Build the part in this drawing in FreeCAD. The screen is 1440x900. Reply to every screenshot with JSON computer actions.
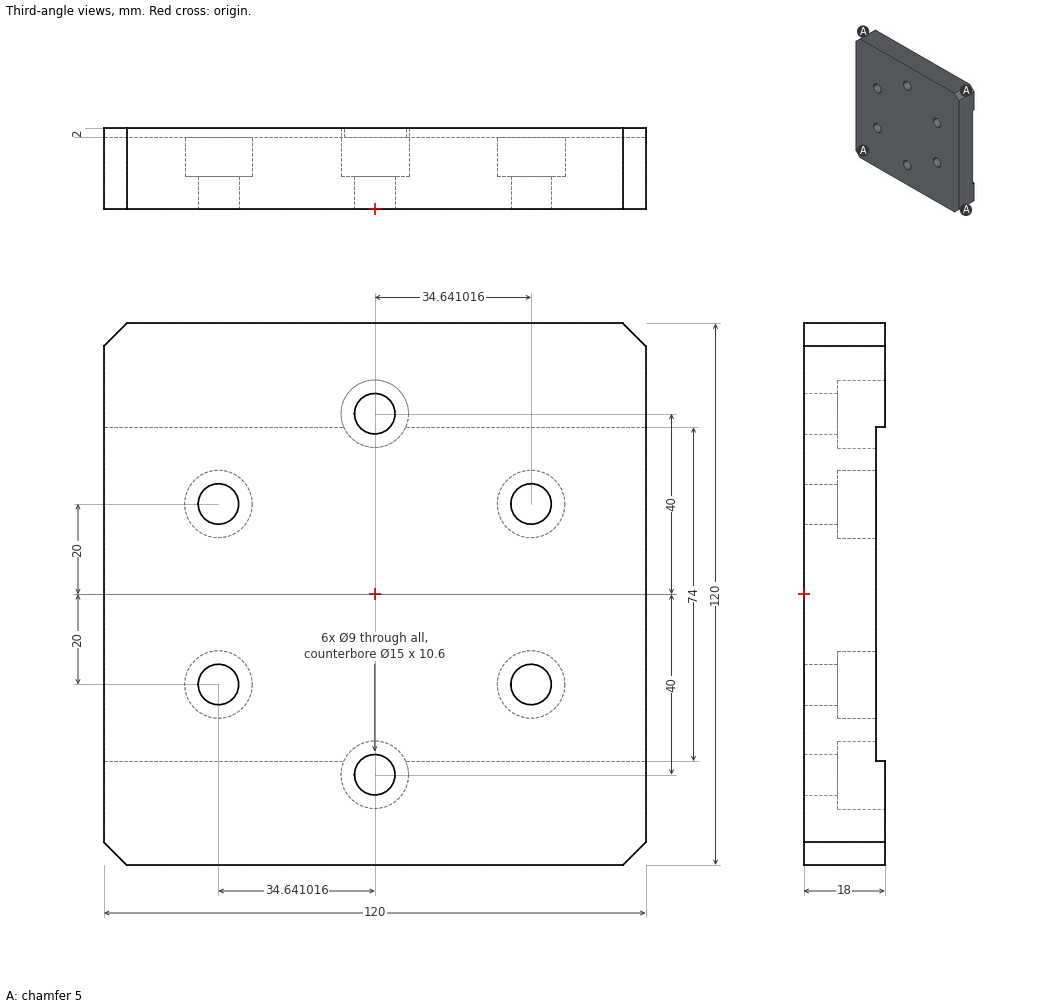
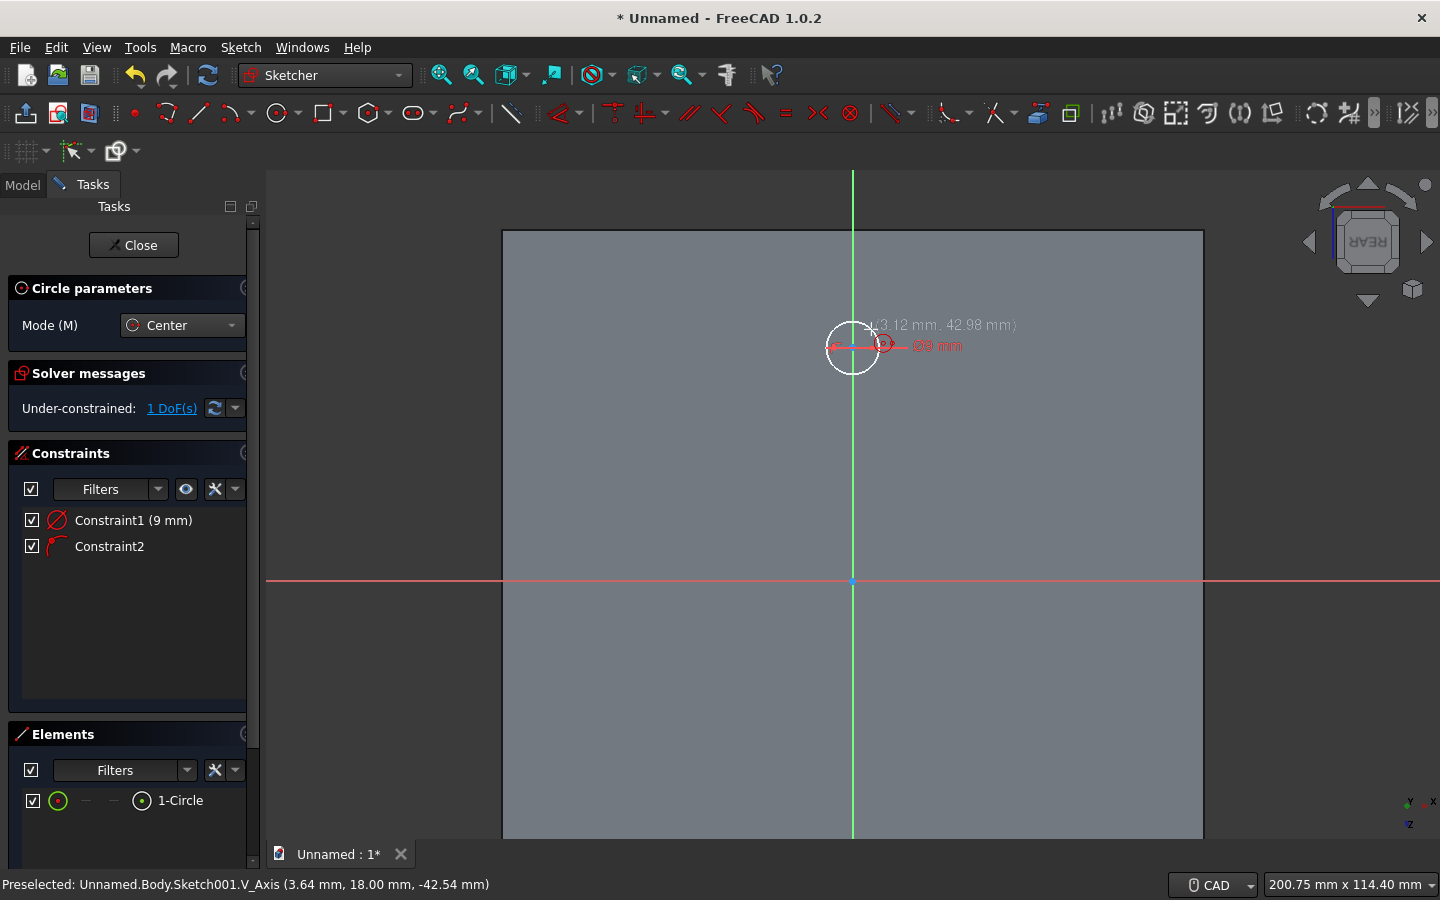
{"action": "left_click", "coordinate": [650, 464]}
{"action": "mouse_move", "coordinate": [669, 446]}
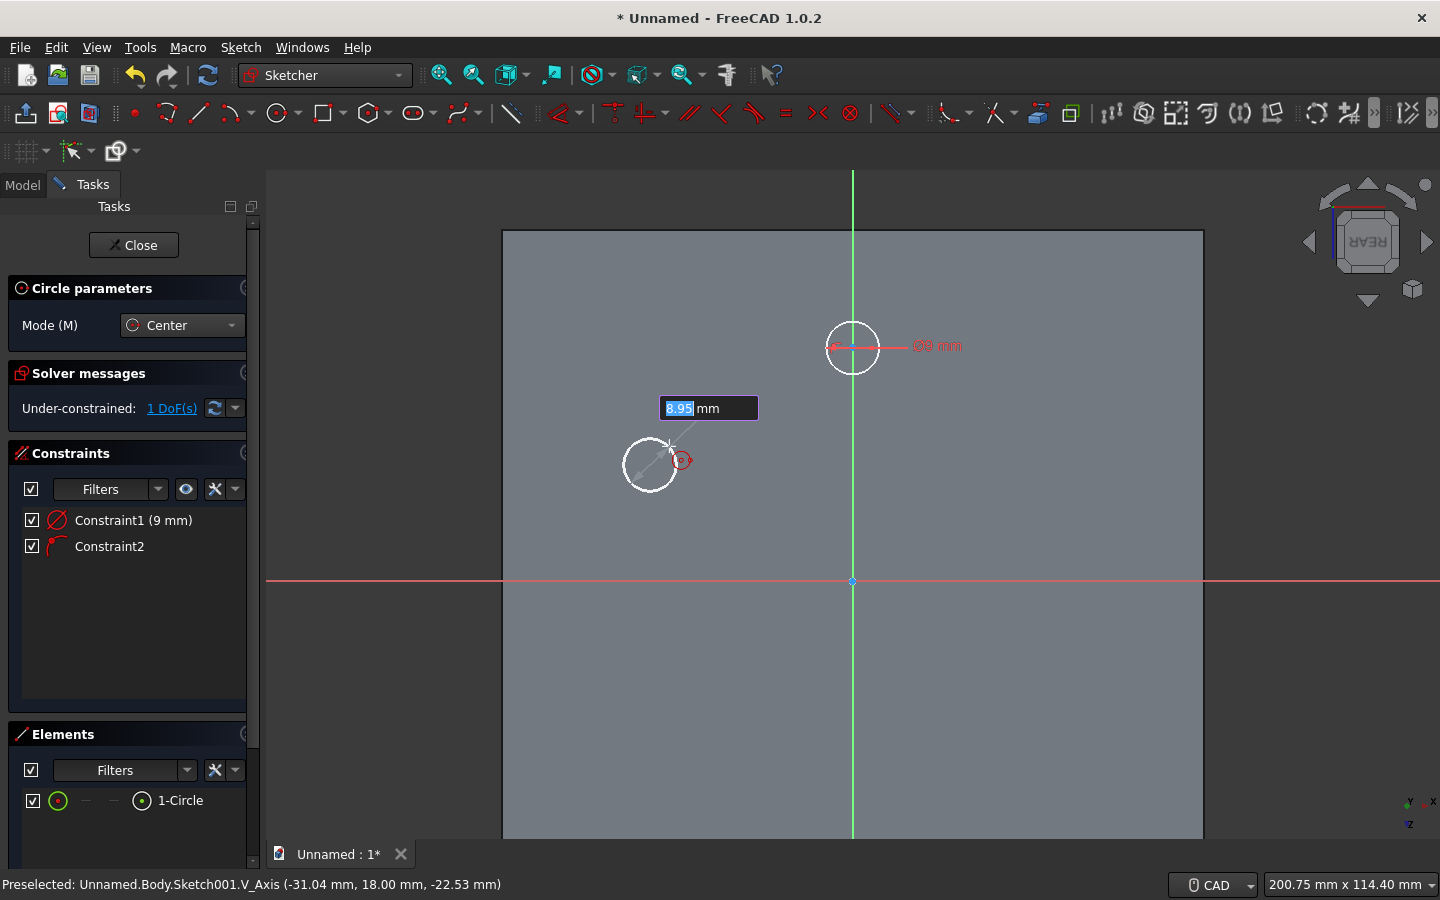
{"action": "type", "text": "9"}
{"action": "key", "text": "Return"}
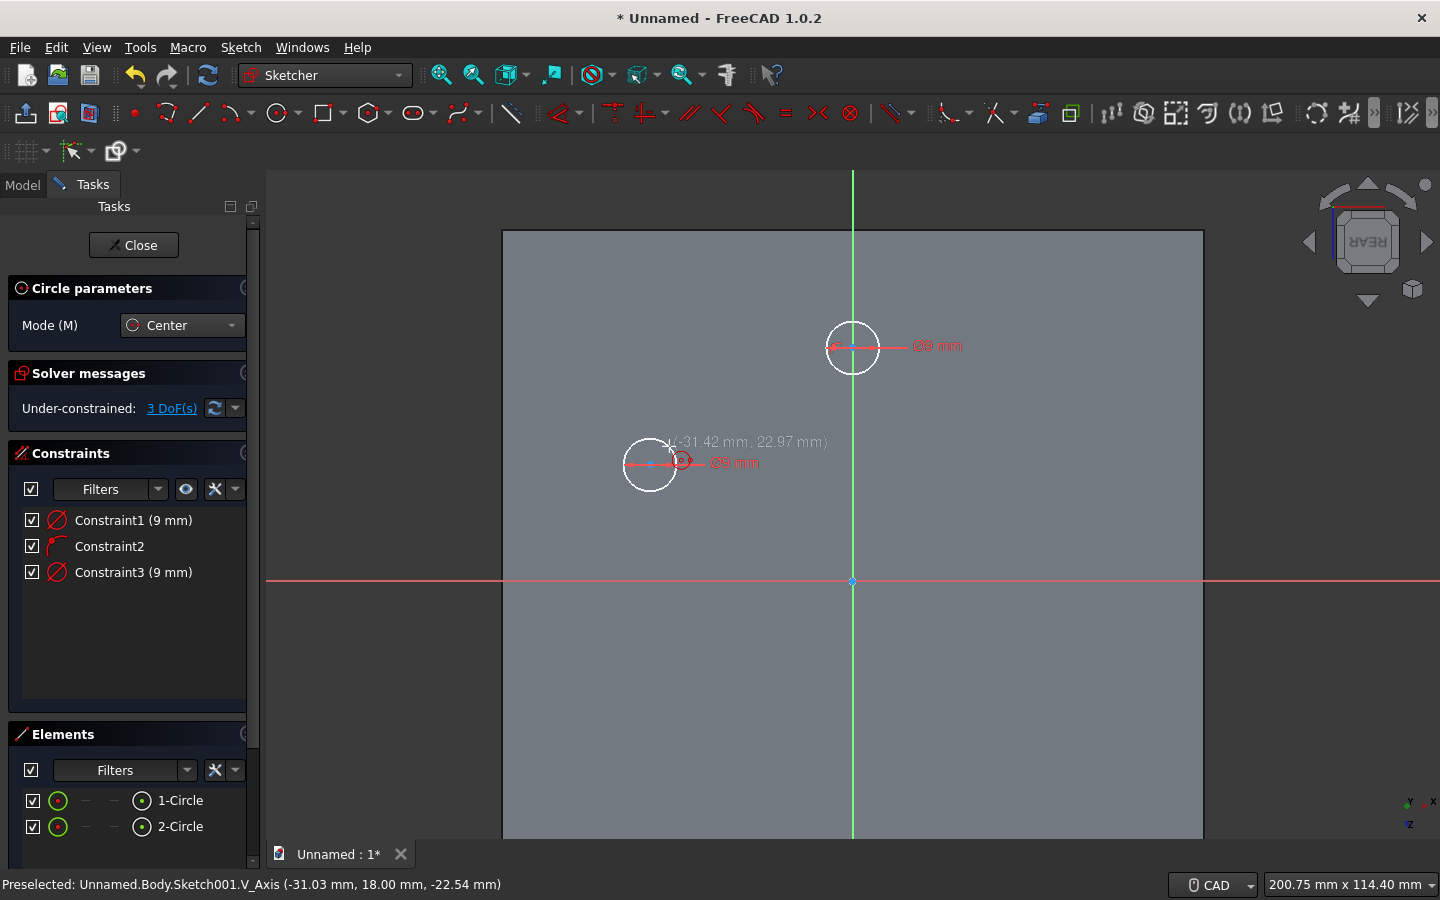
{"action": "left_click", "coordinate": [650, 698]}
{"action": "mouse_move", "coordinate": [669, 680]}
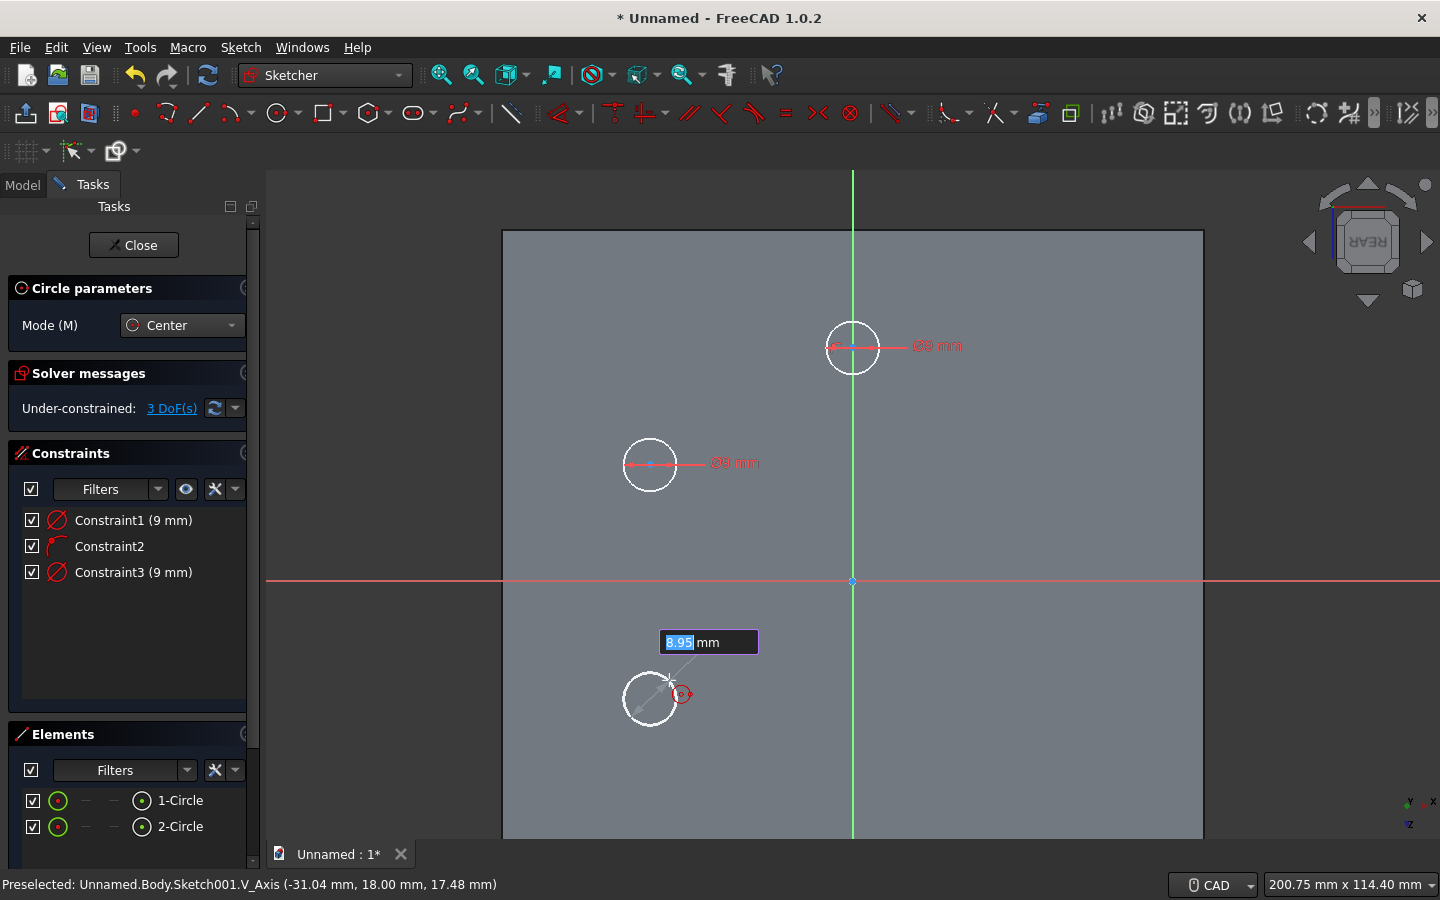
{"action": "type", "text": "9"}
{"action": "key", "text": "Return"}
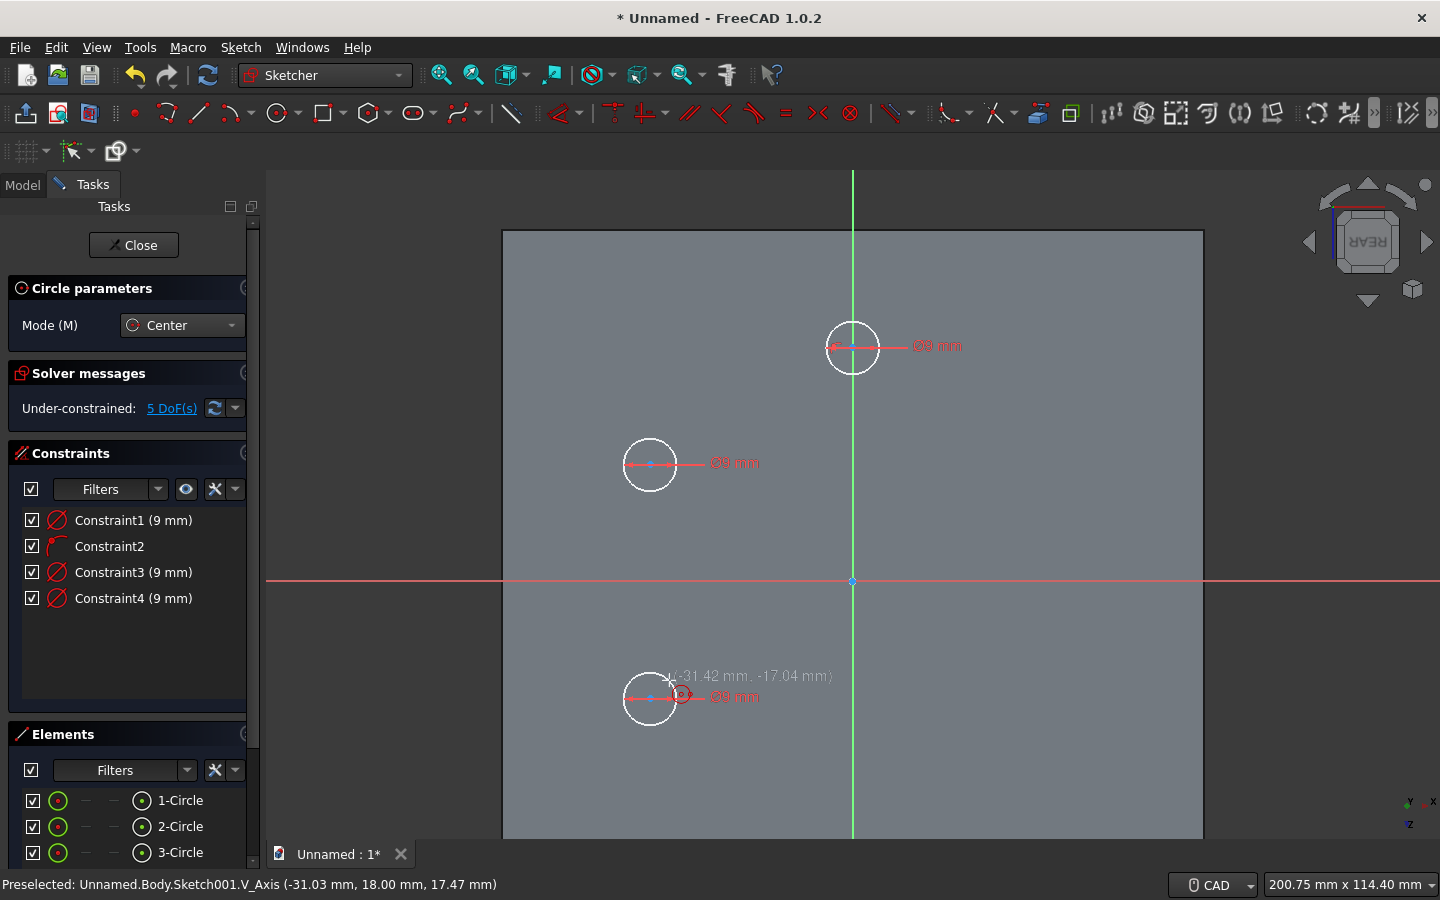
{"action": "scroll", "coordinate": [476, 198], "scroll_direction": "down", "scroll_amount": 1}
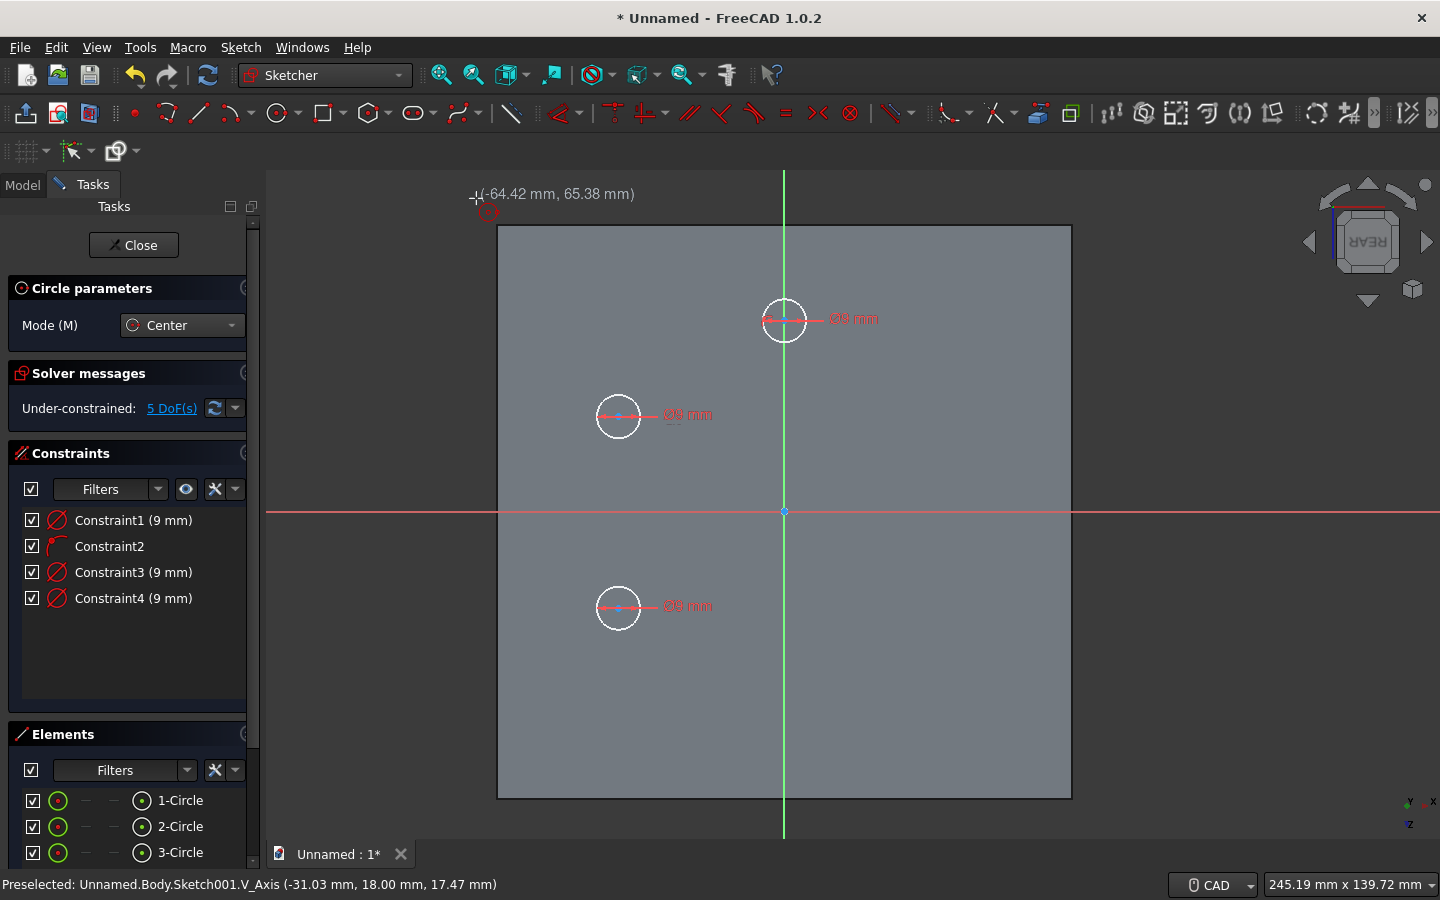
{"action": "left_click", "coordinate": [784, 703]}
{"action": "mouse_move", "coordinate": [800, 688]}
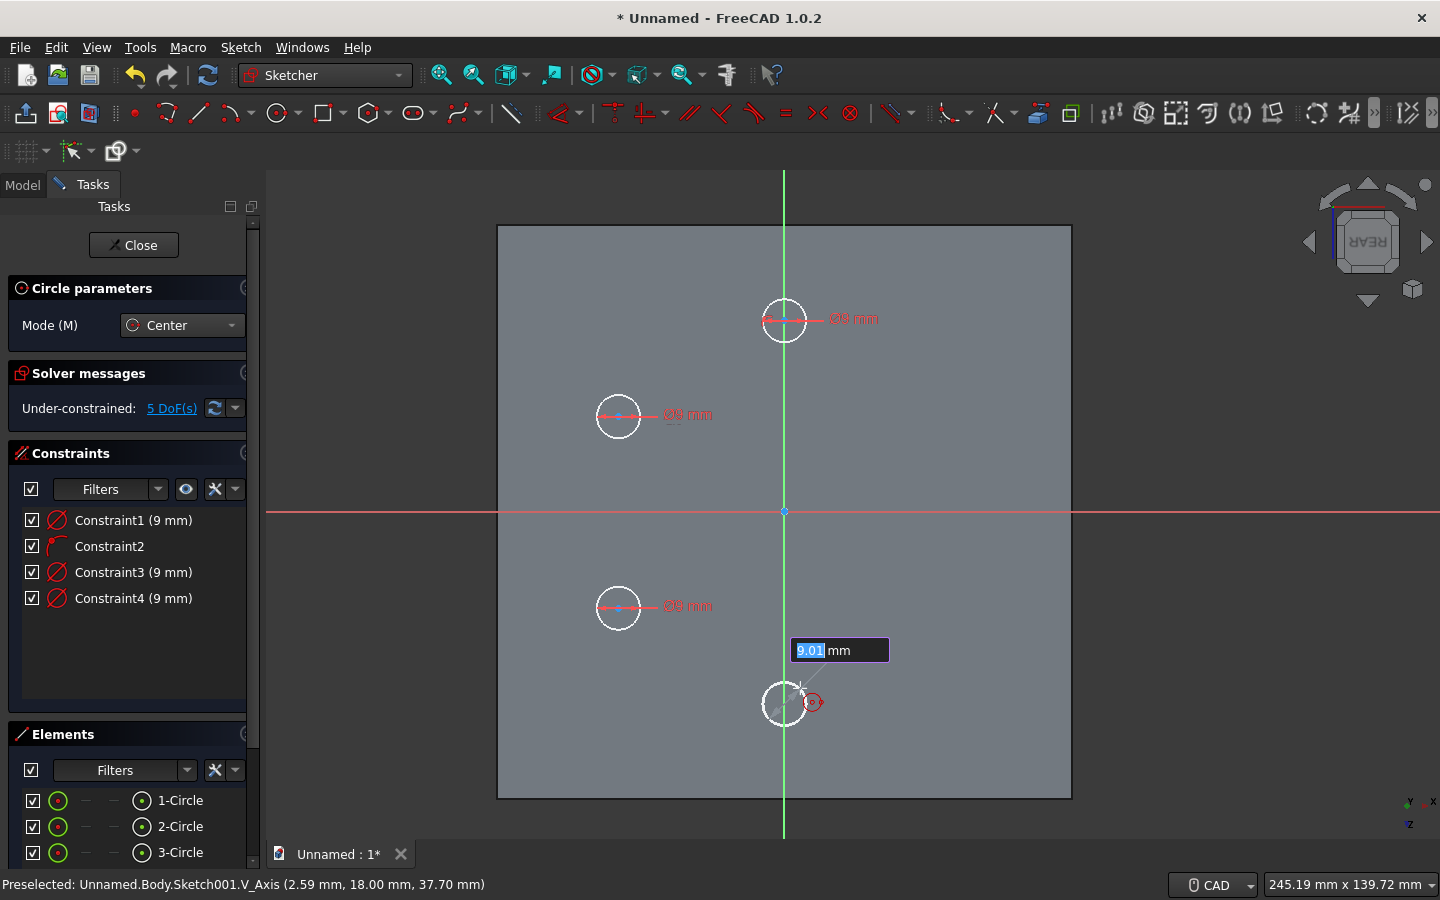
{"action": "type", "text": "9"}
{"action": "key", "text": "Return"}